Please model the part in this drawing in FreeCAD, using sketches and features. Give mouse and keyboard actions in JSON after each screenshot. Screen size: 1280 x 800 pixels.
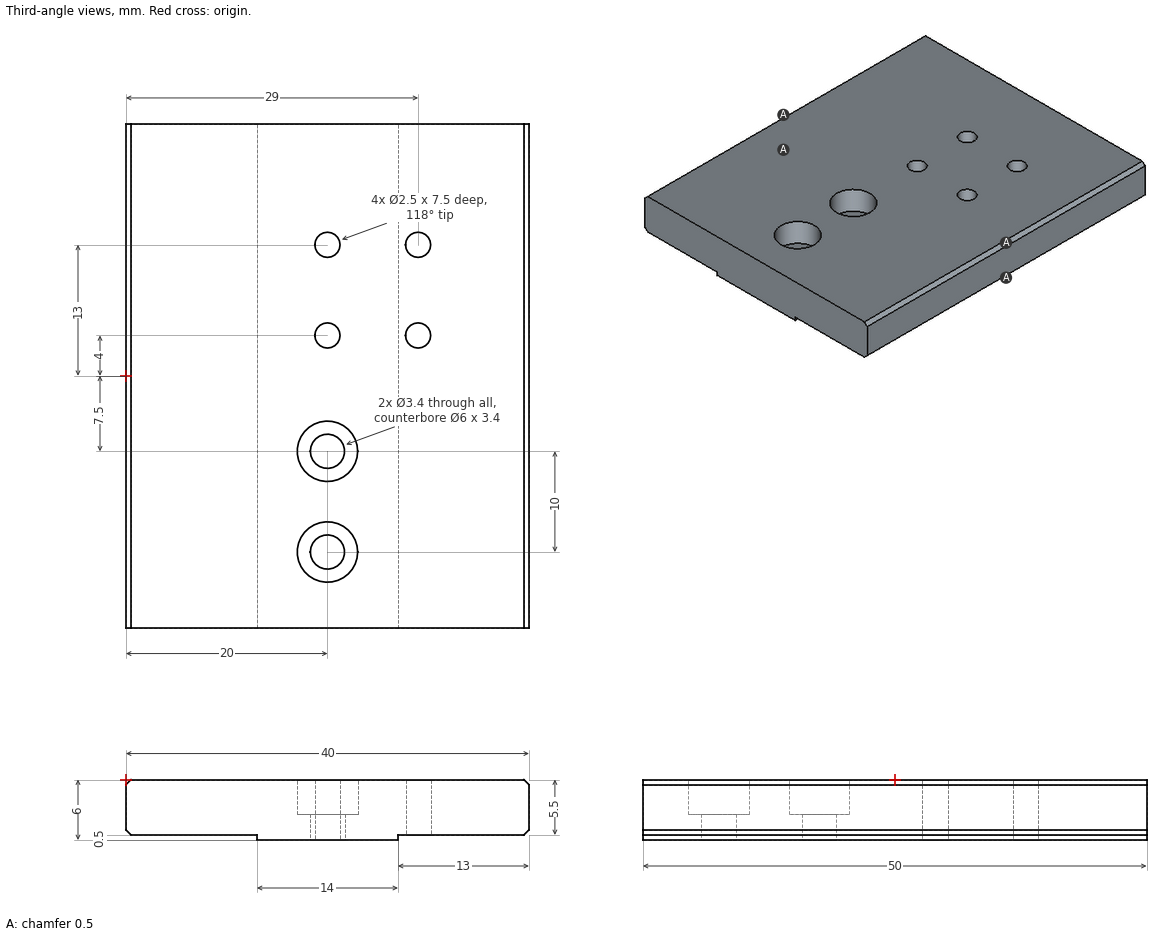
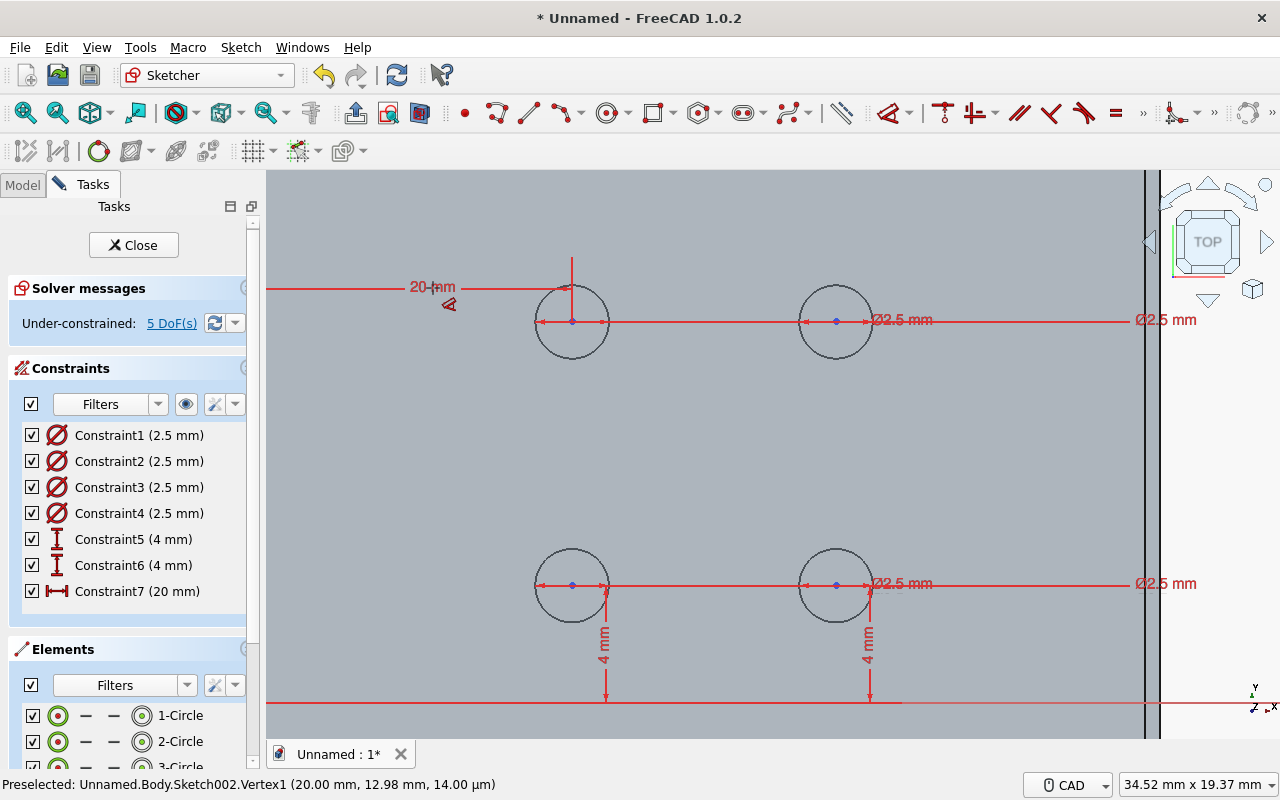
{"action": "left_click", "coordinate": [572, 322]}
{"action": "left_click", "coordinate": [606, 513]}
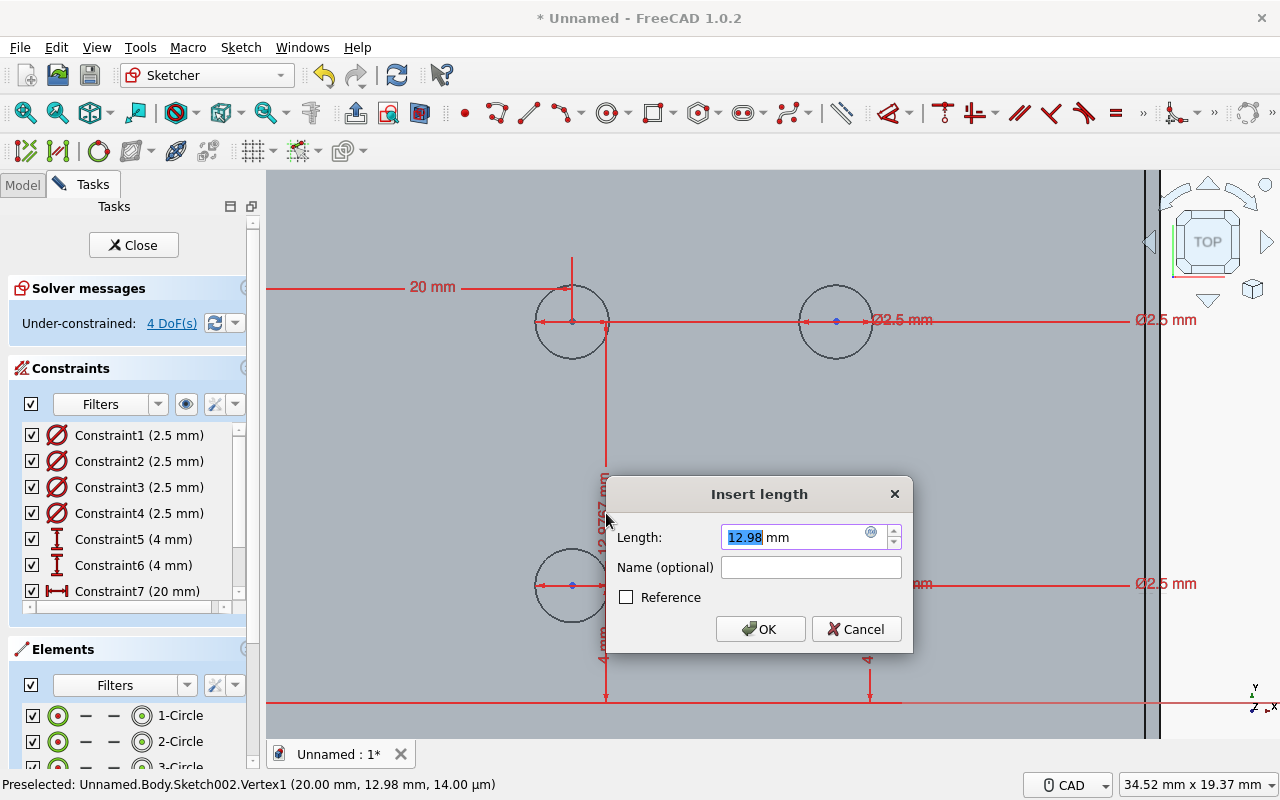
{"action": "type", "text": "13"}
{"action": "key", "text": "Return"}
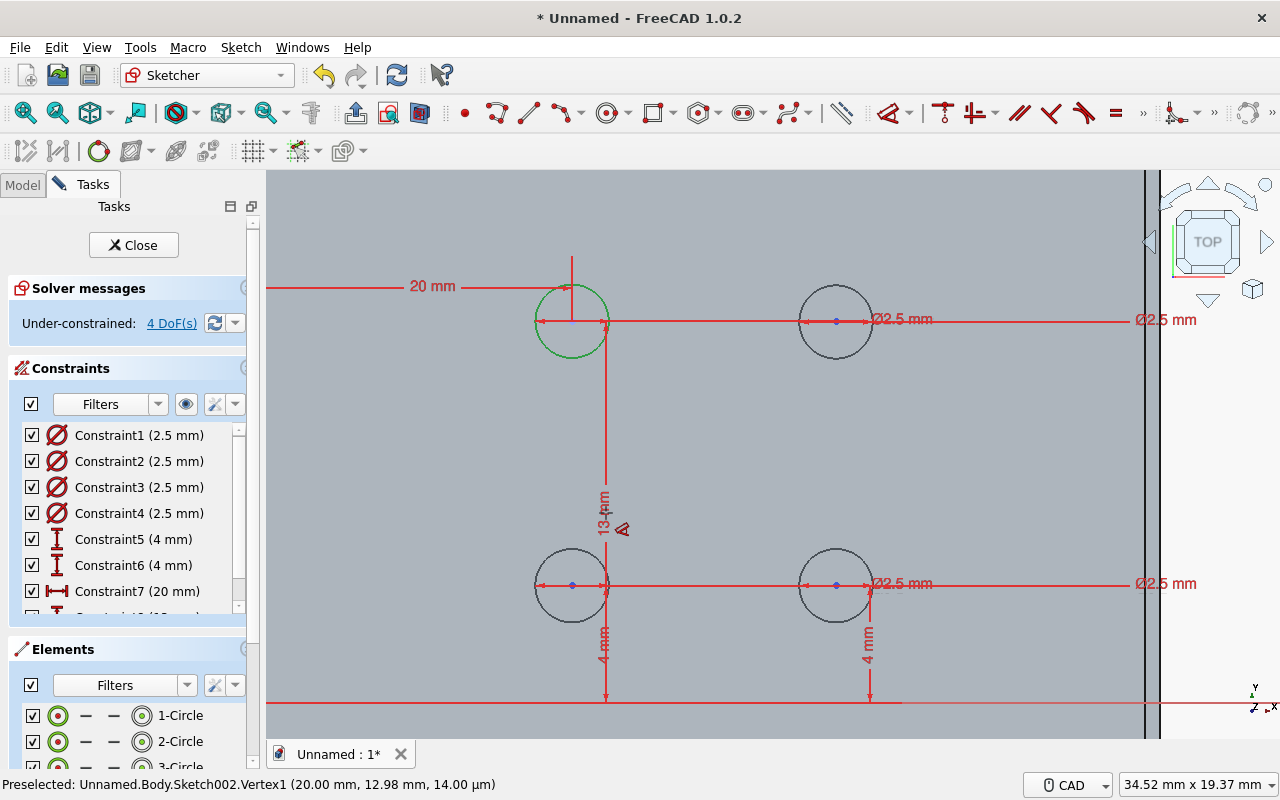
{"action": "left_click", "coordinate": [836, 322]}
{"action": "left_click", "coordinate": [690, 288]}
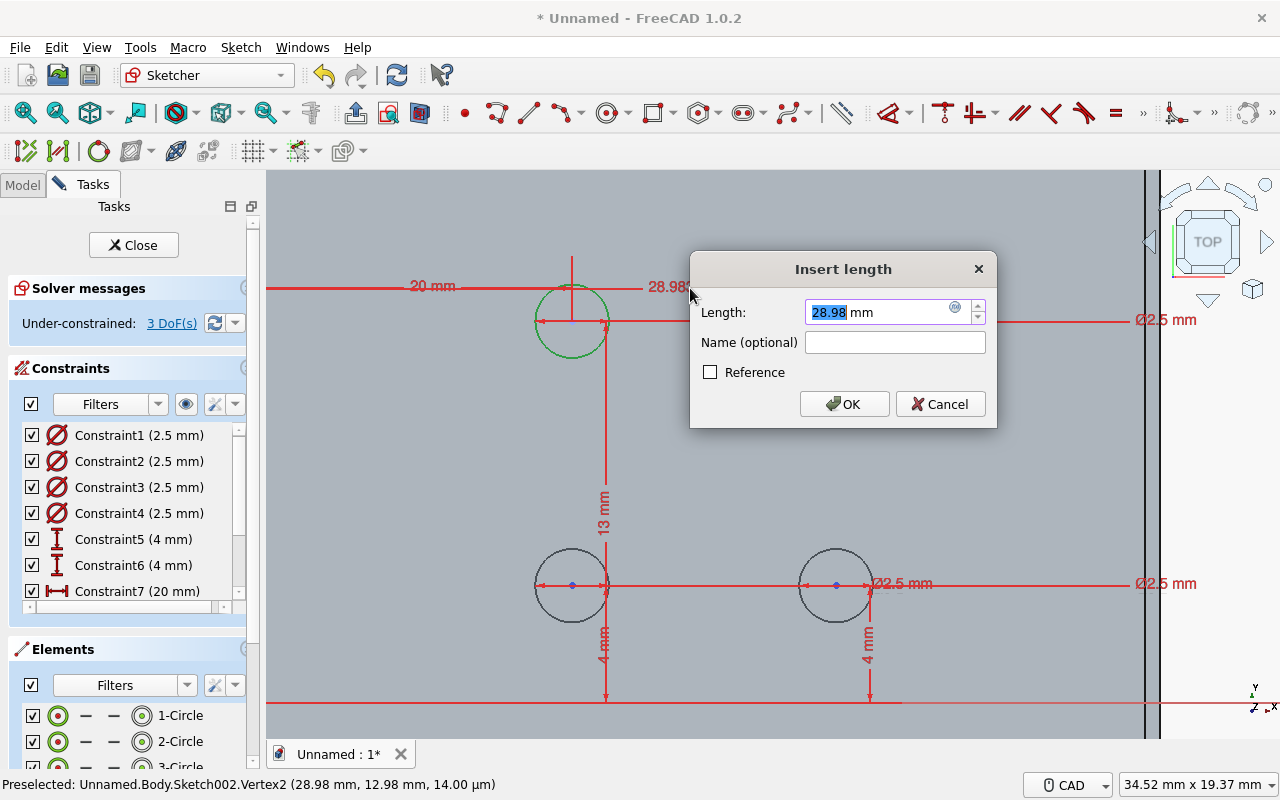
{"action": "type", "text": "29"}
{"action": "key", "text": "Return"}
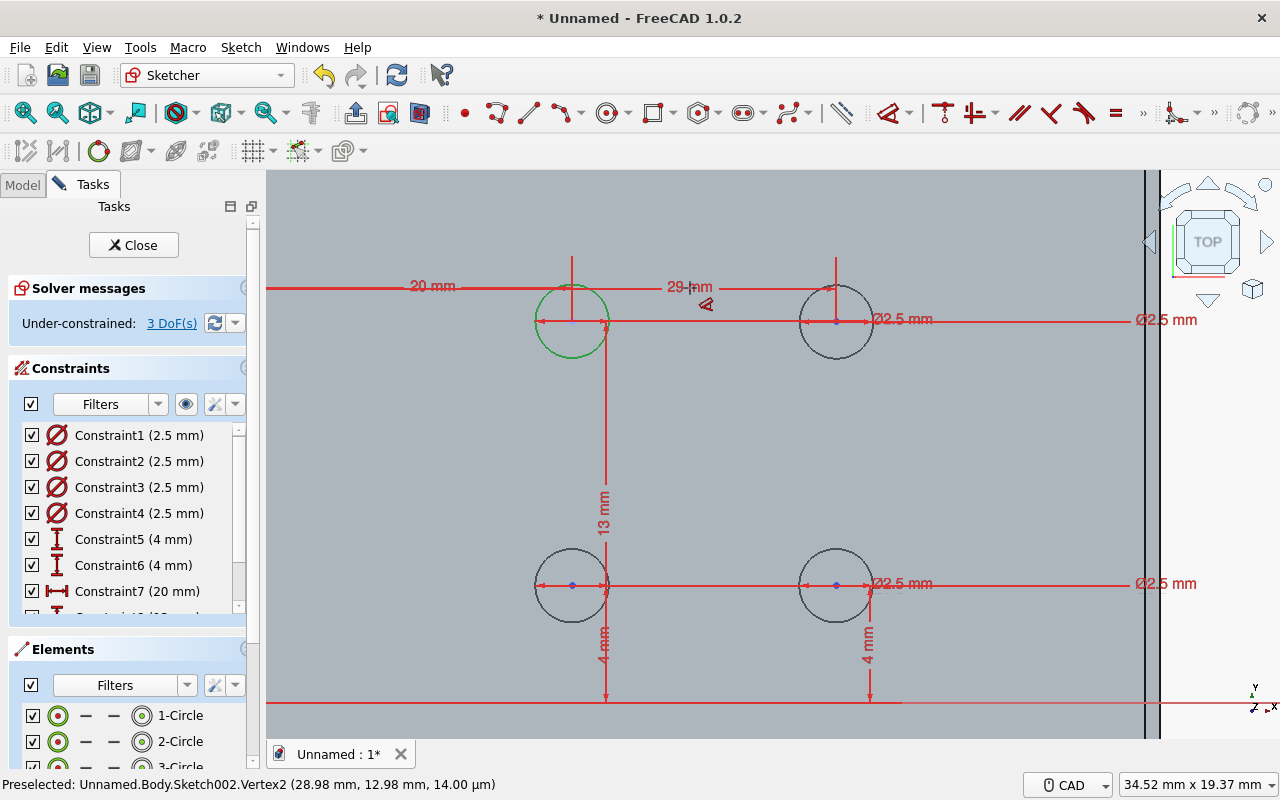
{"action": "left_click", "coordinate": [836, 322]}
{"action": "left_click", "coordinate": [870, 513]}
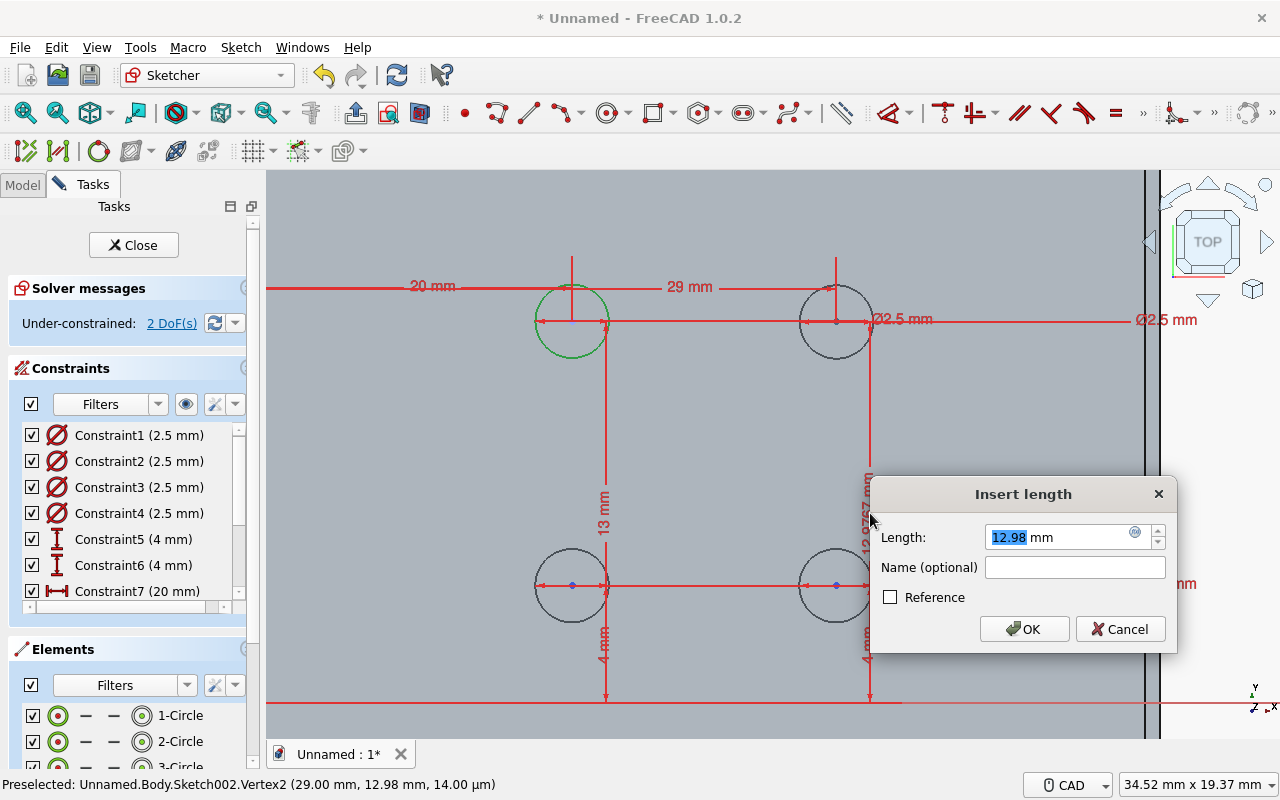
{"action": "type", "text": "13"}
{"action": "key", "text": "Return"}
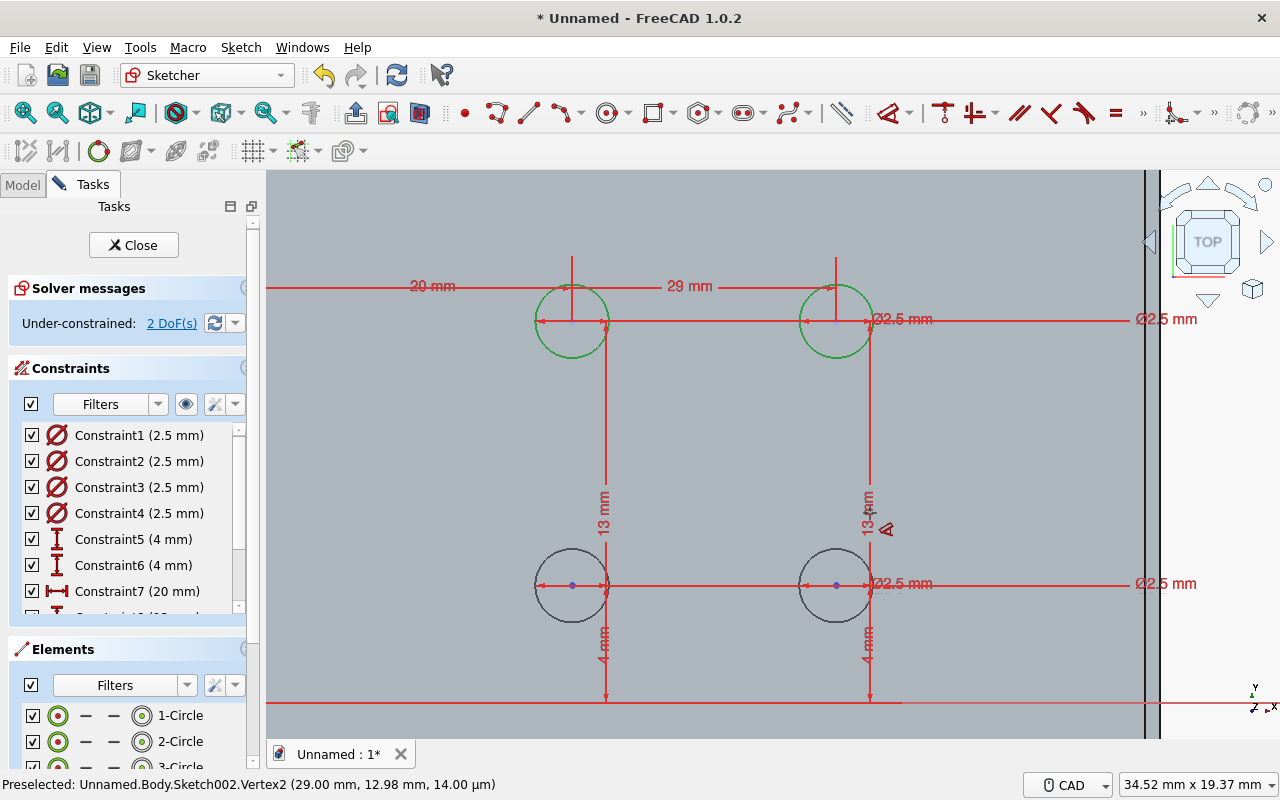
{"action": "left_click", "coordinate": [572, 586]}
{"action": "left_click", "coordinate": [433, 552]}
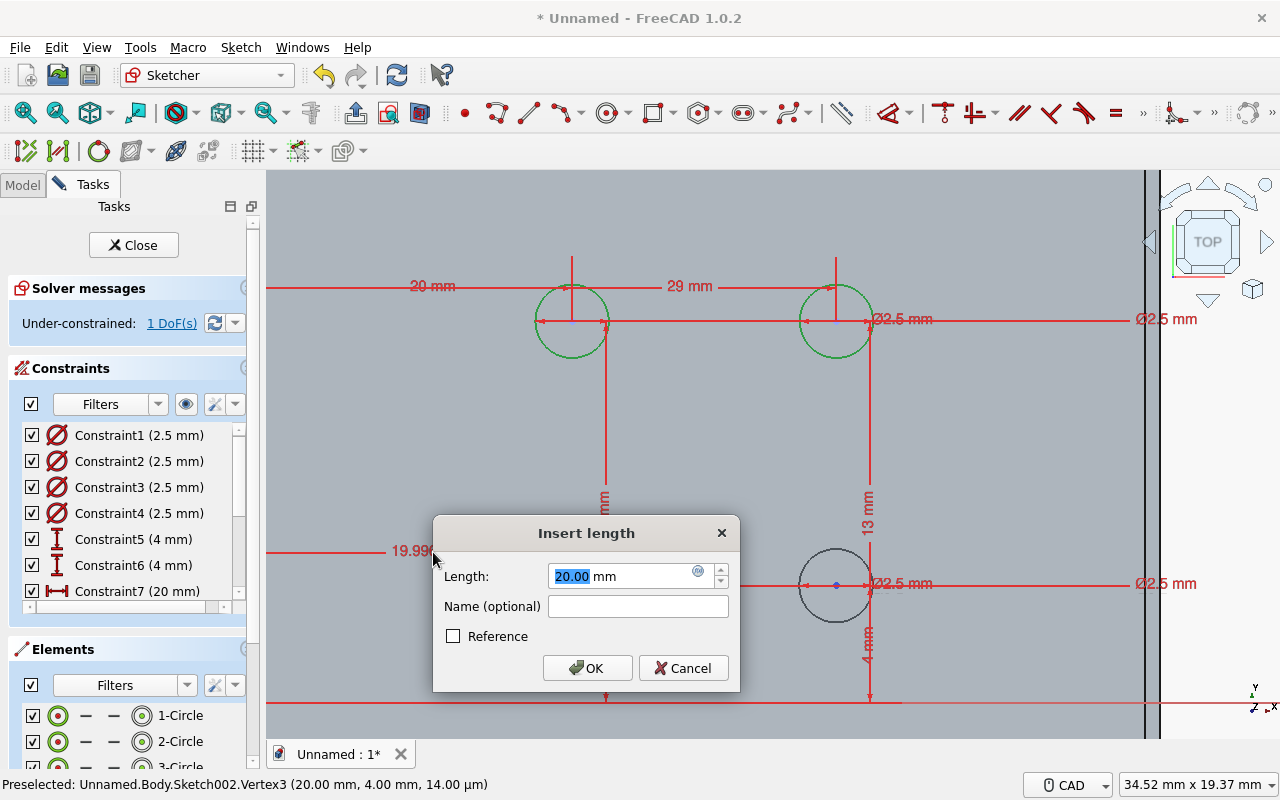
{"action": "type", "text": "20"}
{"action": "key", "text": "Return"}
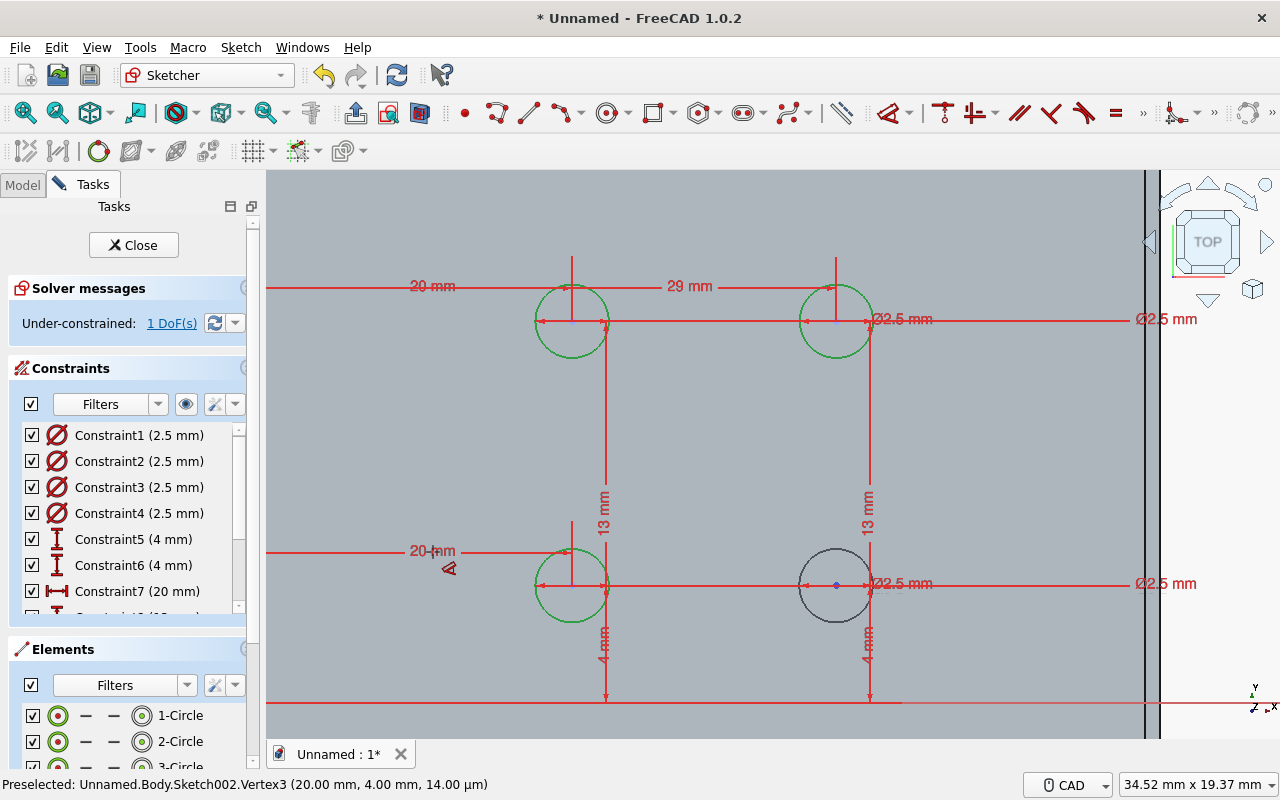
{"action": "left_click", "coordinate": [836, 586]}
{"action": "left_click", "coordinate": [690, 552]}